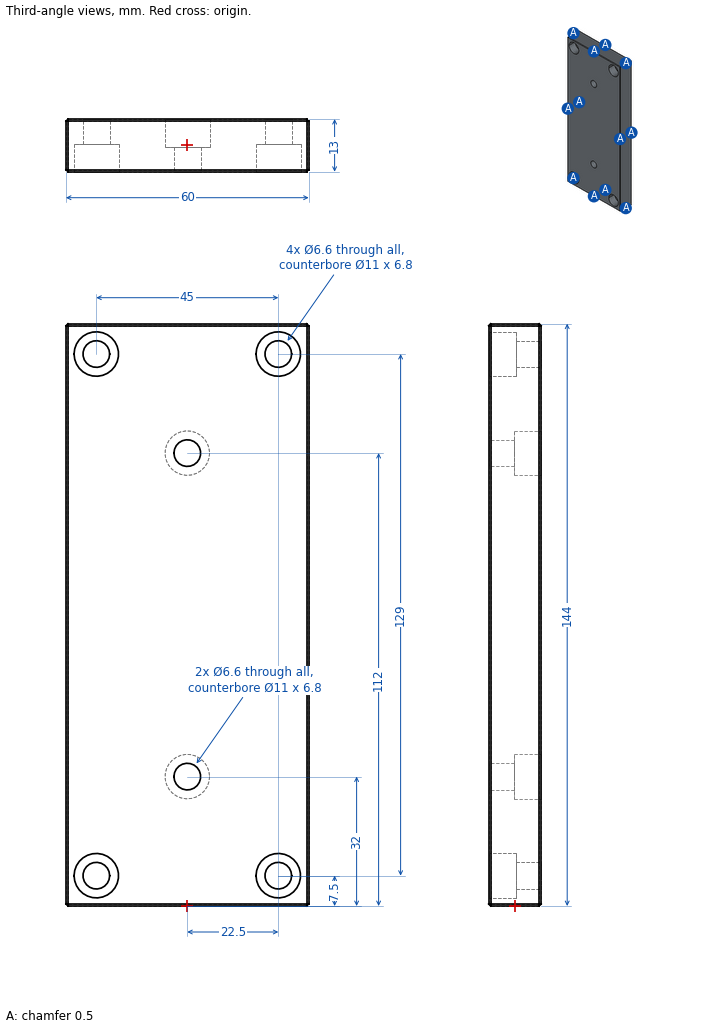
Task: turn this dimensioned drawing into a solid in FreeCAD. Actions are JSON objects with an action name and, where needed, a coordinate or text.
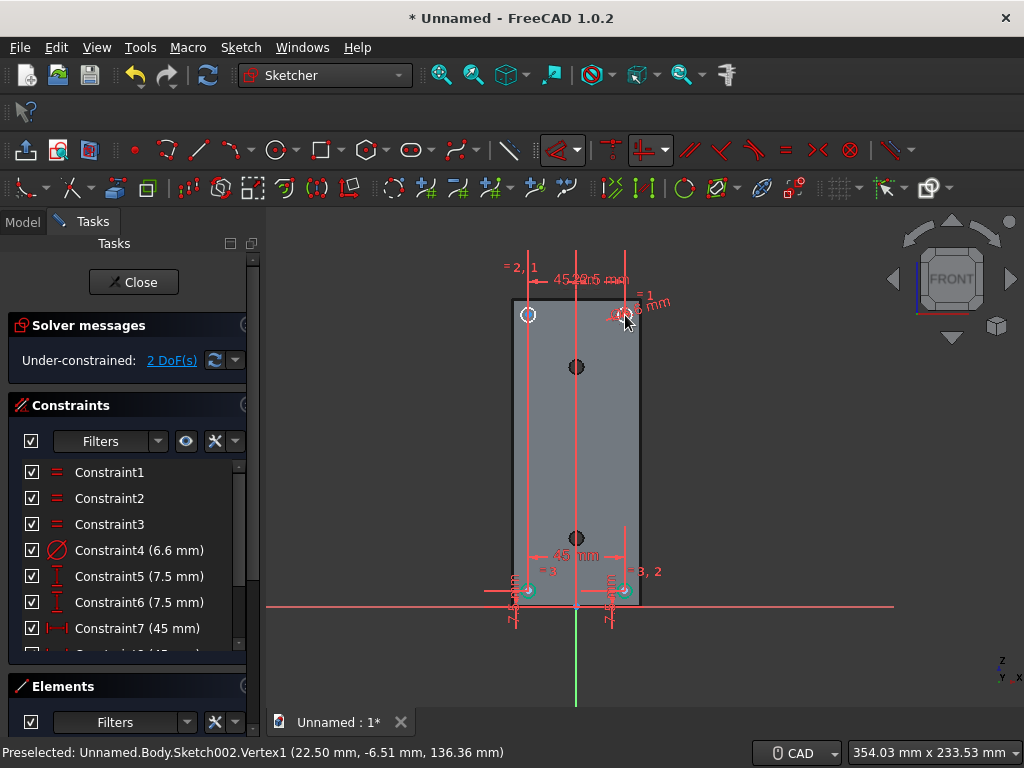
{"action": "left_click", "coordinate": [625, 591]}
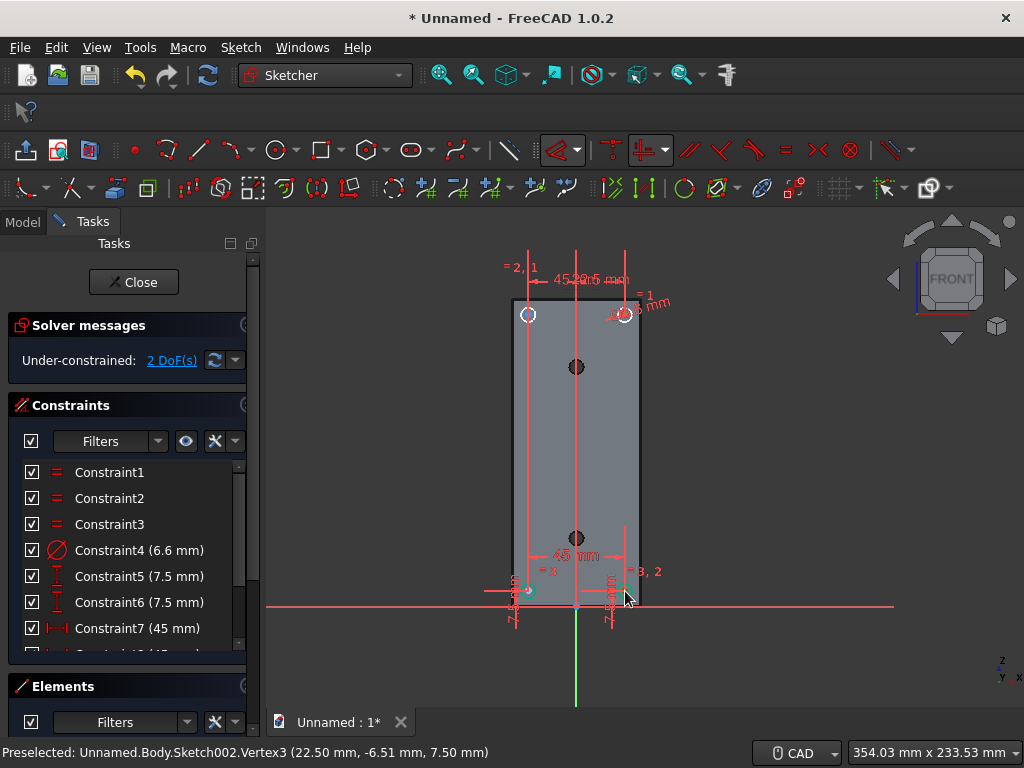
{"action": "key", "text": "i"}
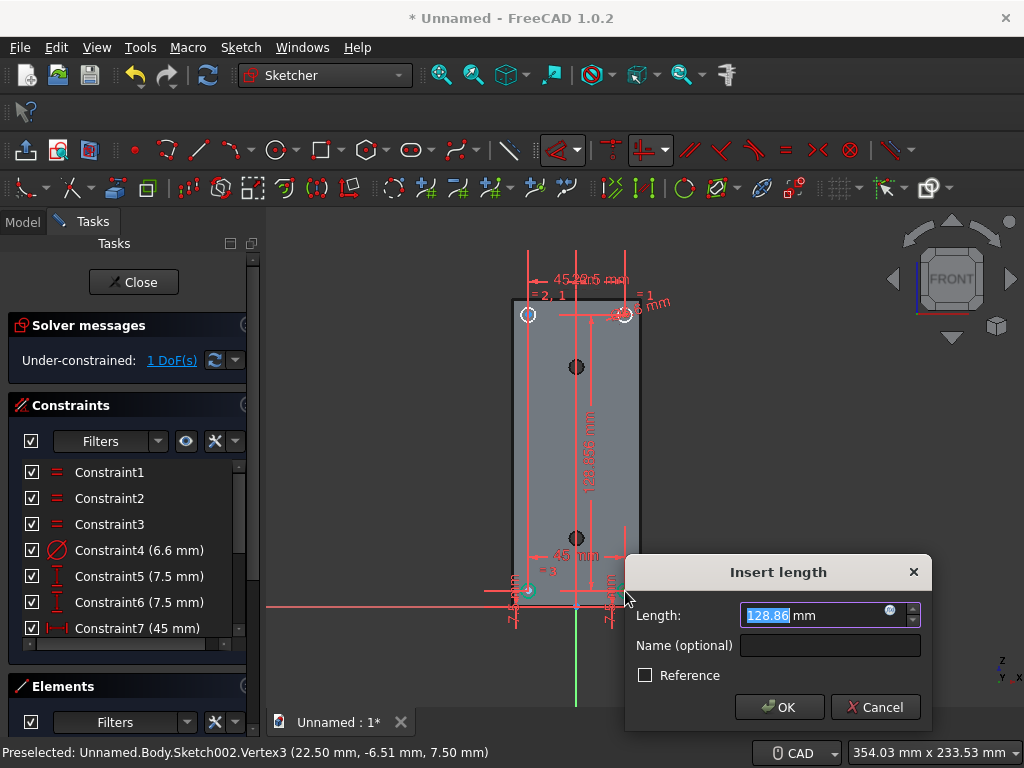
{"action": "type", "text": "129"}
{"action": "key", "text": "Return"}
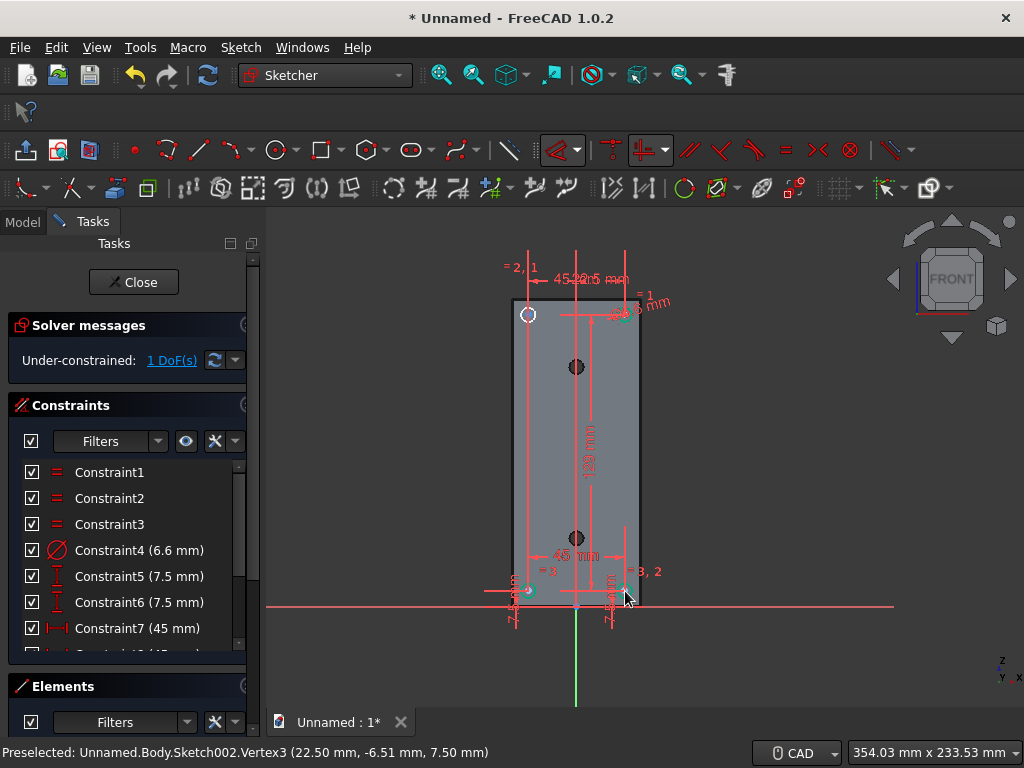
{"action": "left_click", "coordinate": [528, 315]}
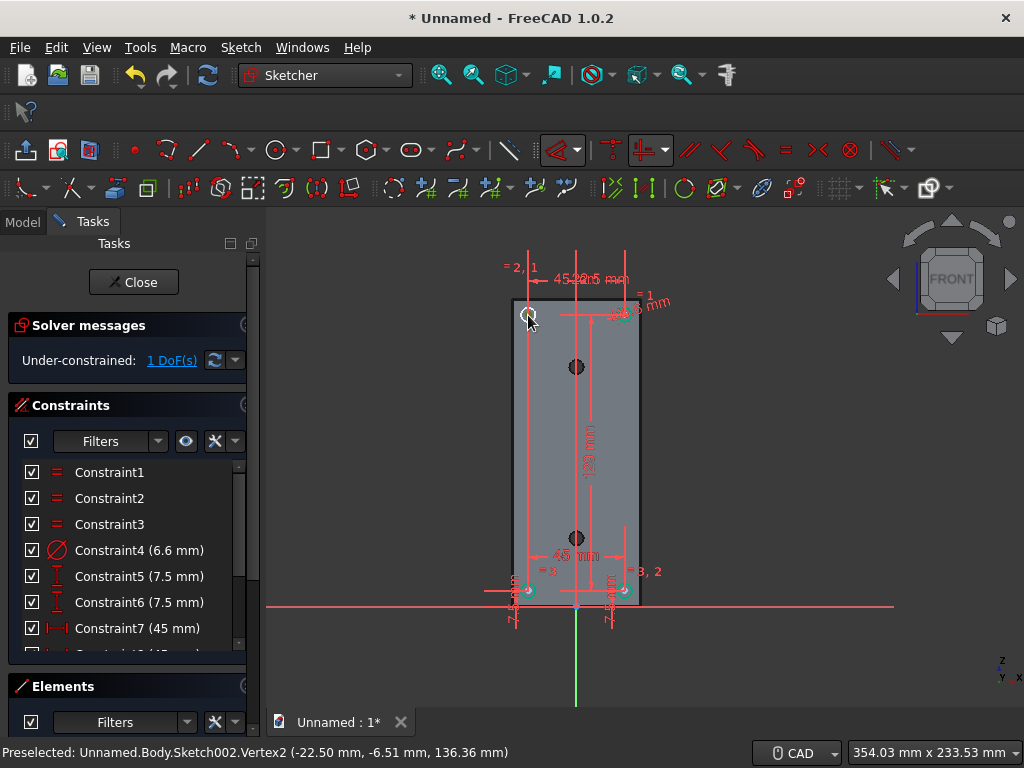
{"action": "left_click", "coordinate": [625, 591]}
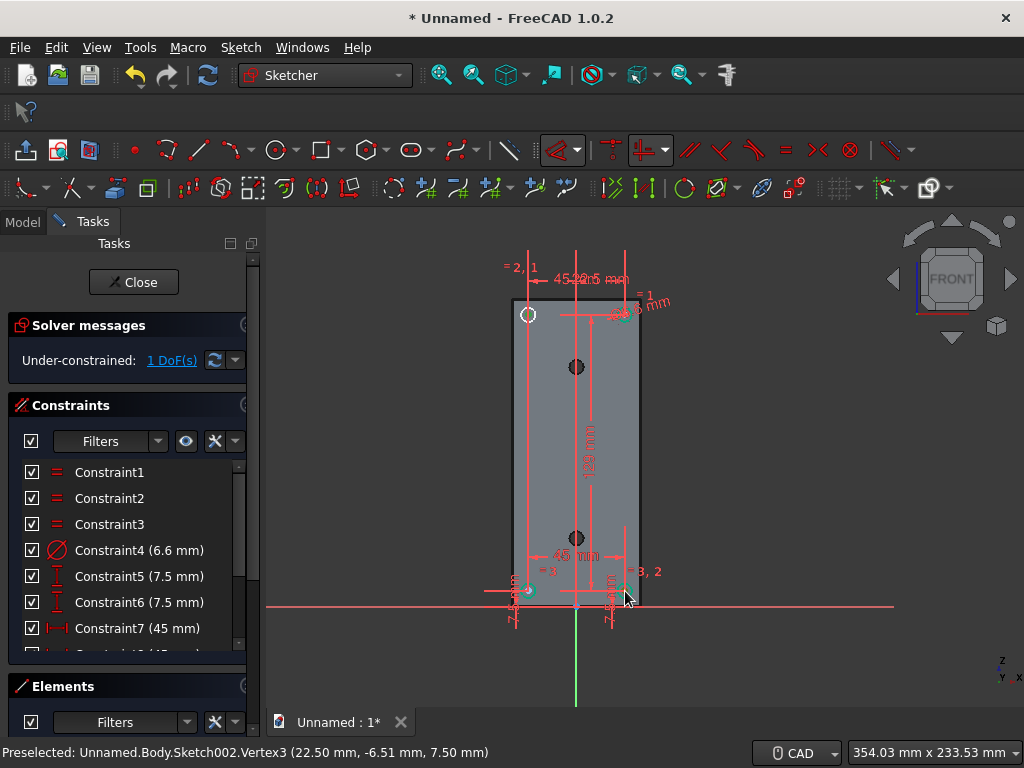
{"action": "left_click", "coordinate": [580, 150]}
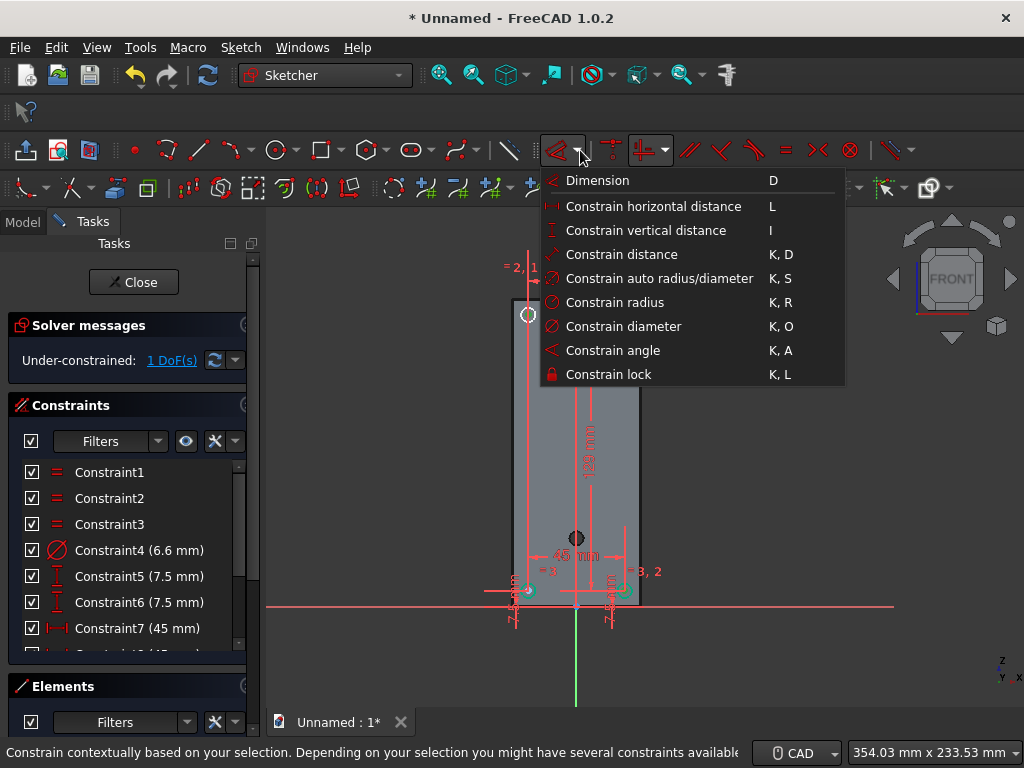
{"action": "left_click", "coordinate": [693, 230]}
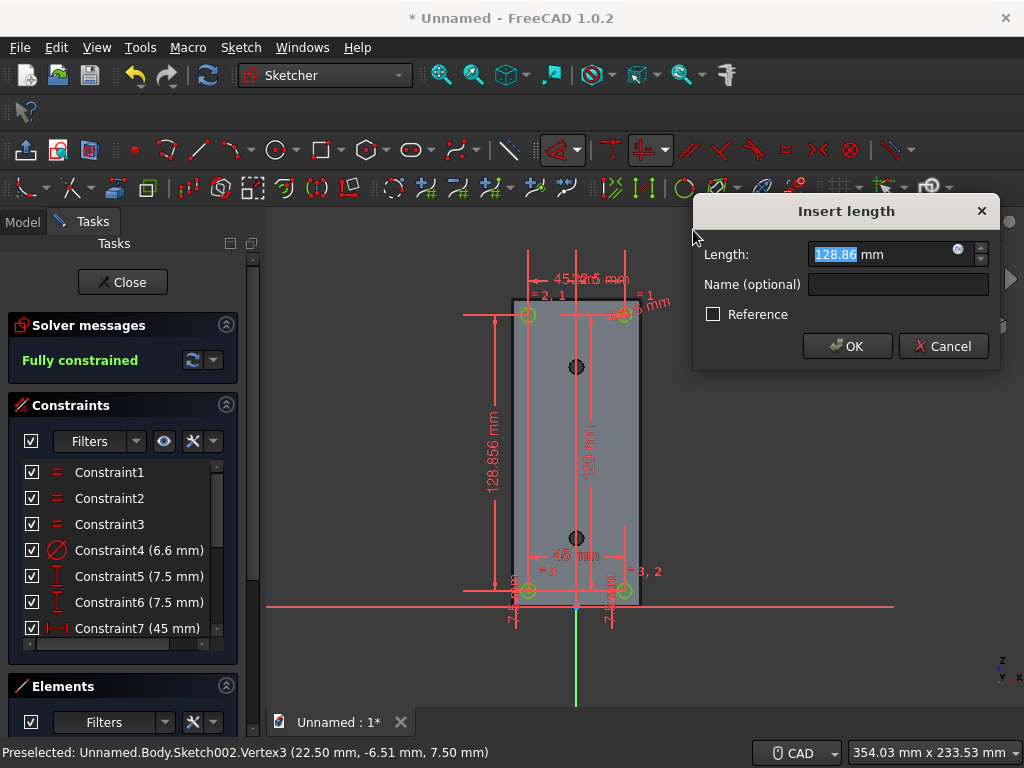
{"action": "type", "text": "129"}
{"action": "key", "text": "Return"}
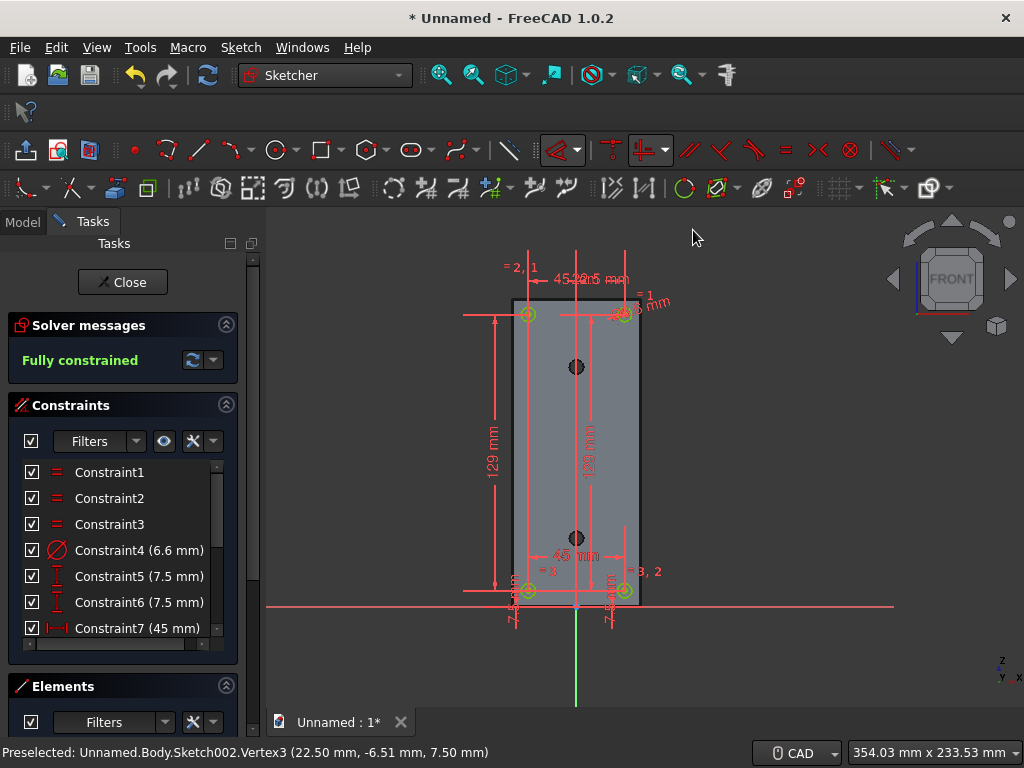
{"action": "left_click", "coordinate": [123, 282]}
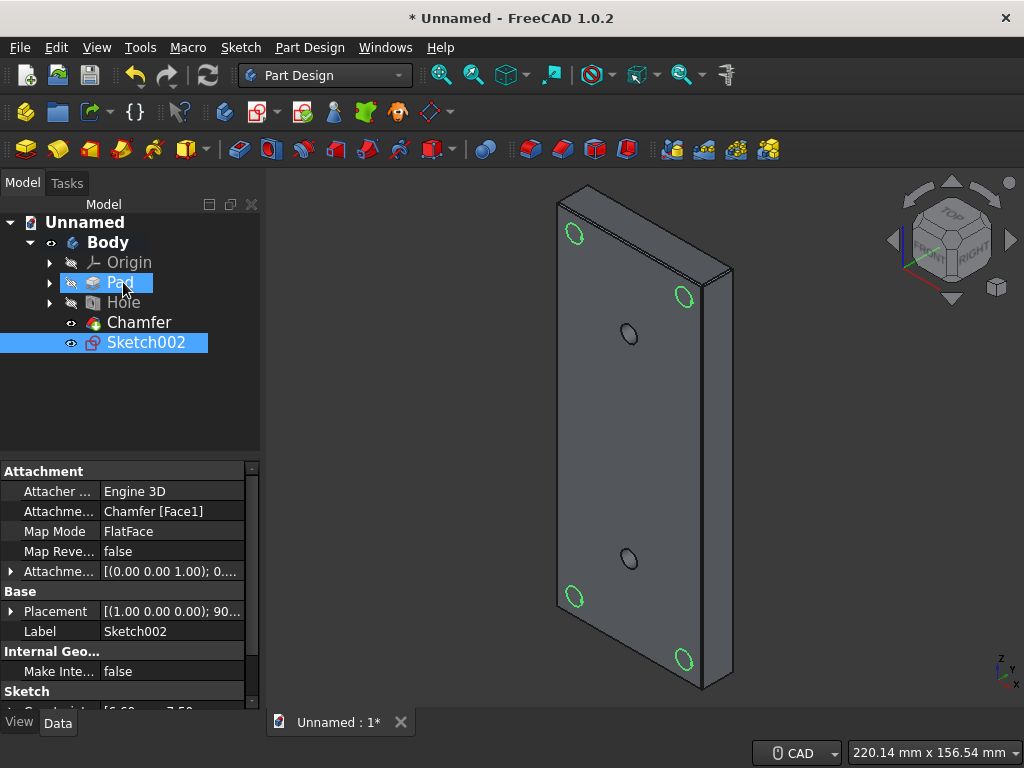
{"action": "left_click", "coordinate": [272, 150]}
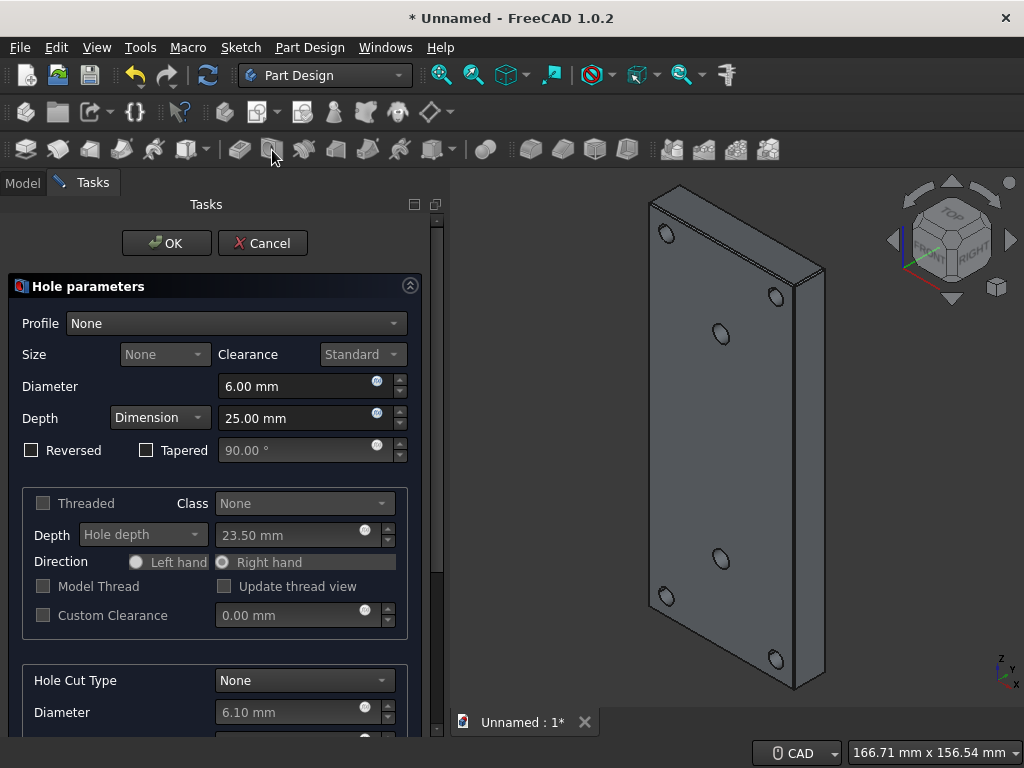
{"action": "triple_click", "coordinate": [305, 386]}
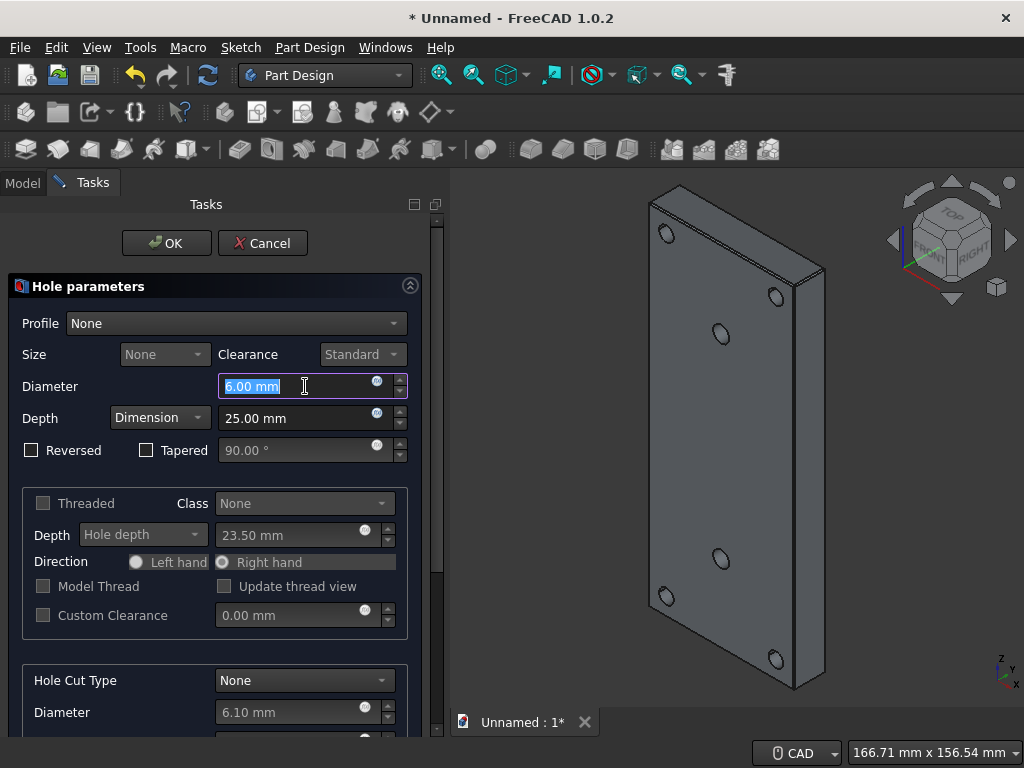
{"action": "type", "text": "6.6"}
{"action": "key", "text": "Tab"}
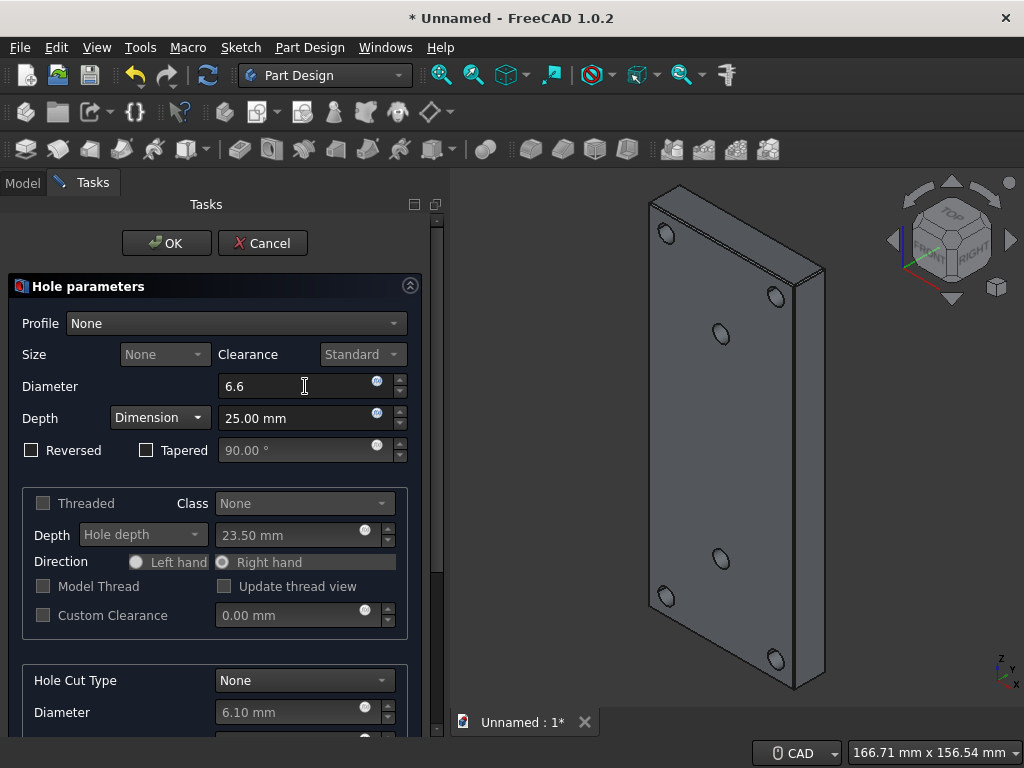
{"action": "left_click", "coordinate": [161, 418]}